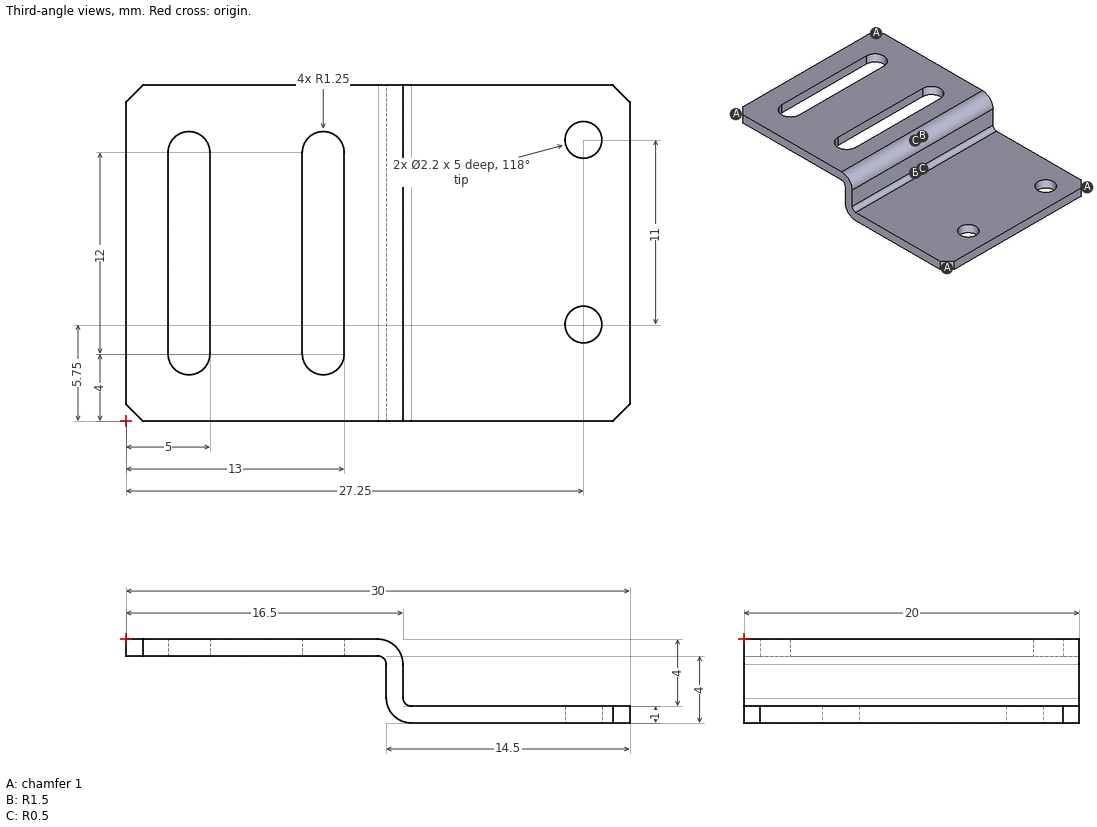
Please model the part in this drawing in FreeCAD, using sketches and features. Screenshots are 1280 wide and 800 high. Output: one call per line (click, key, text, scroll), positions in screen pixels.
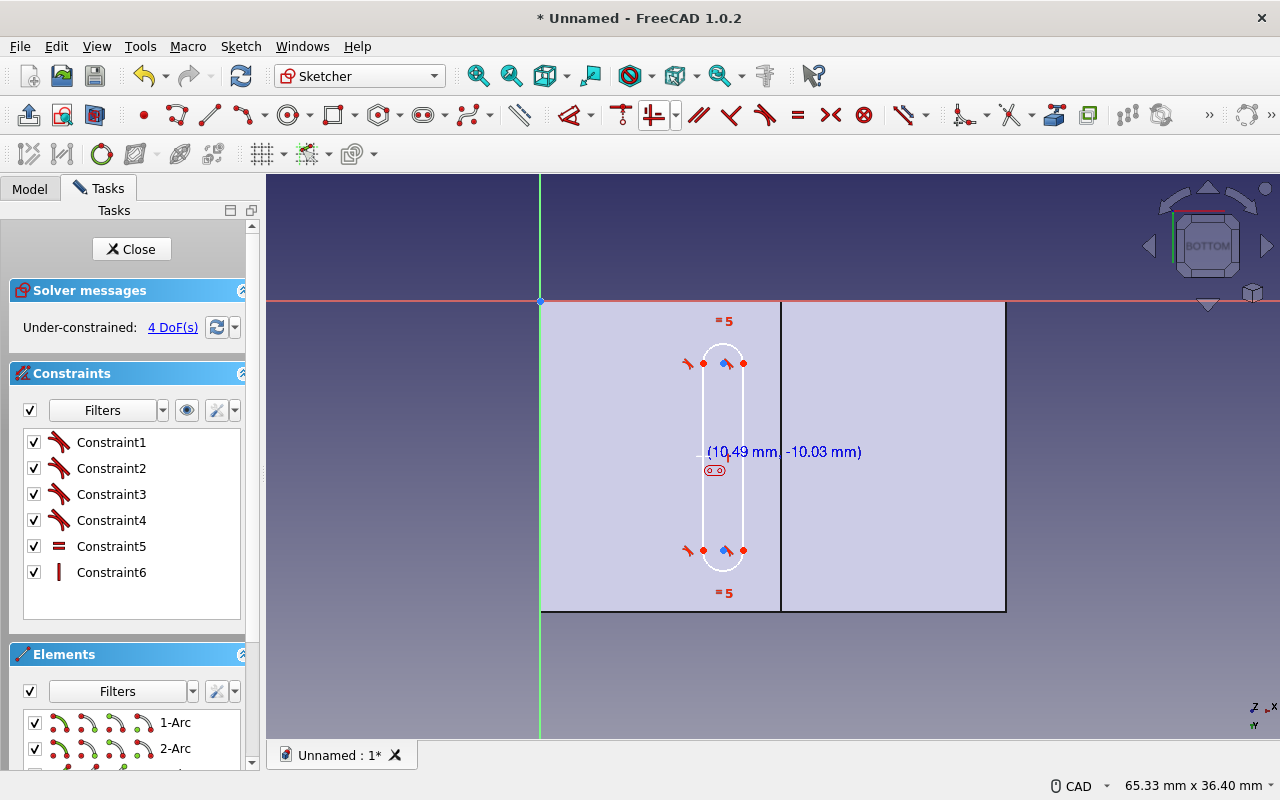
click(598, 550)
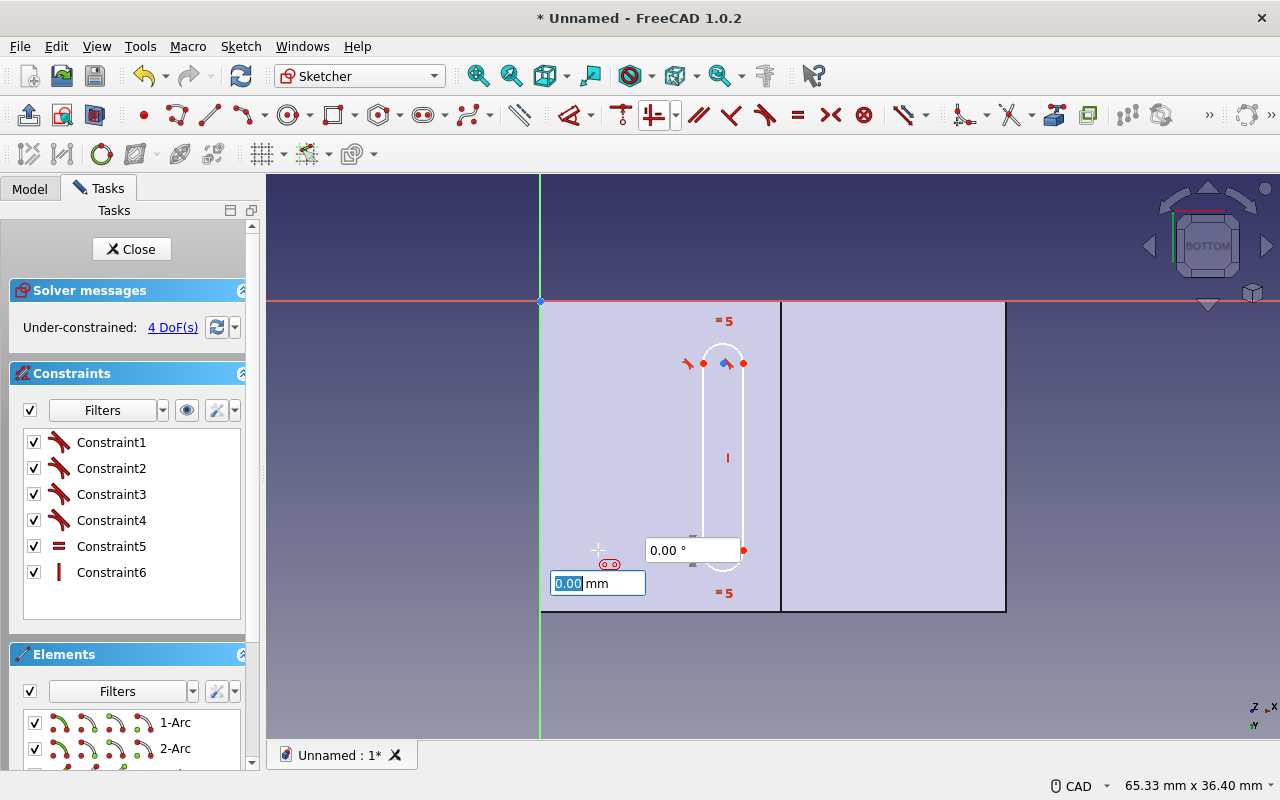
click(598, 363)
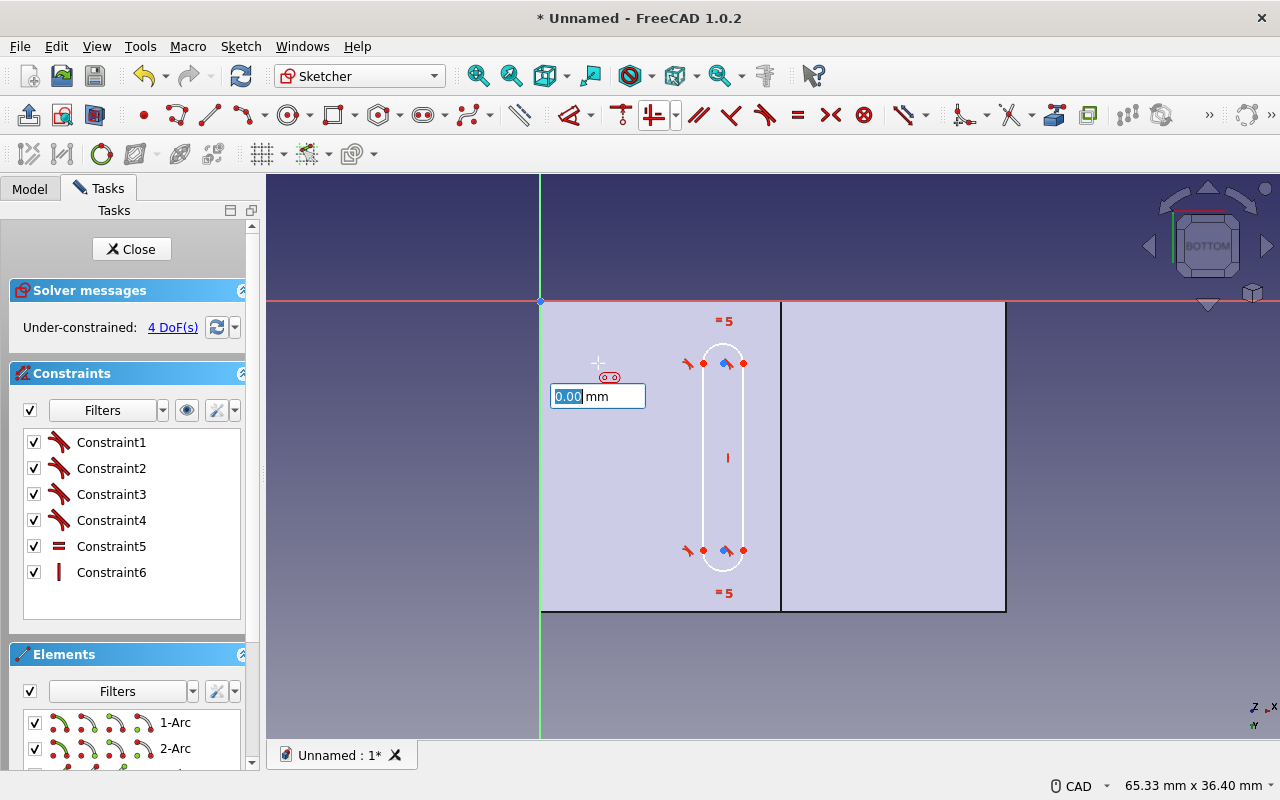
click(618, 456)
key(Escape)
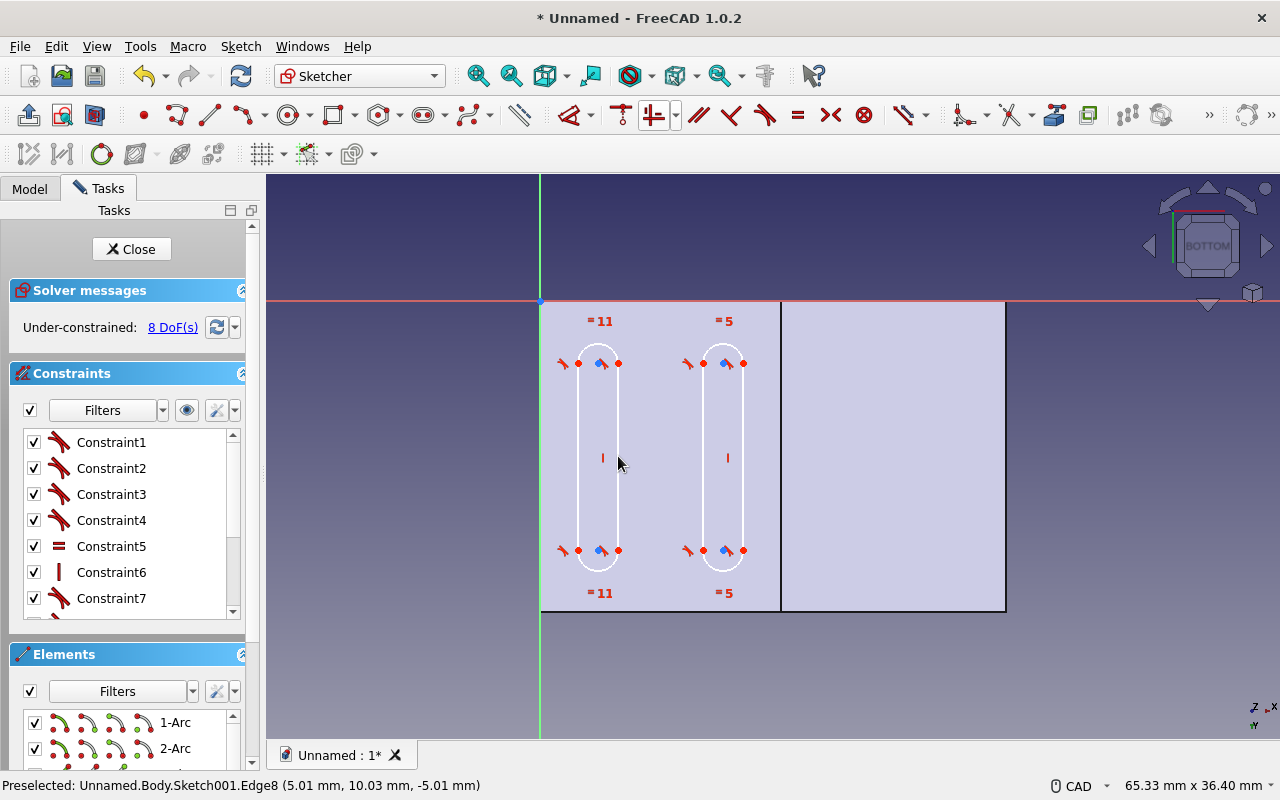
click(711, 567)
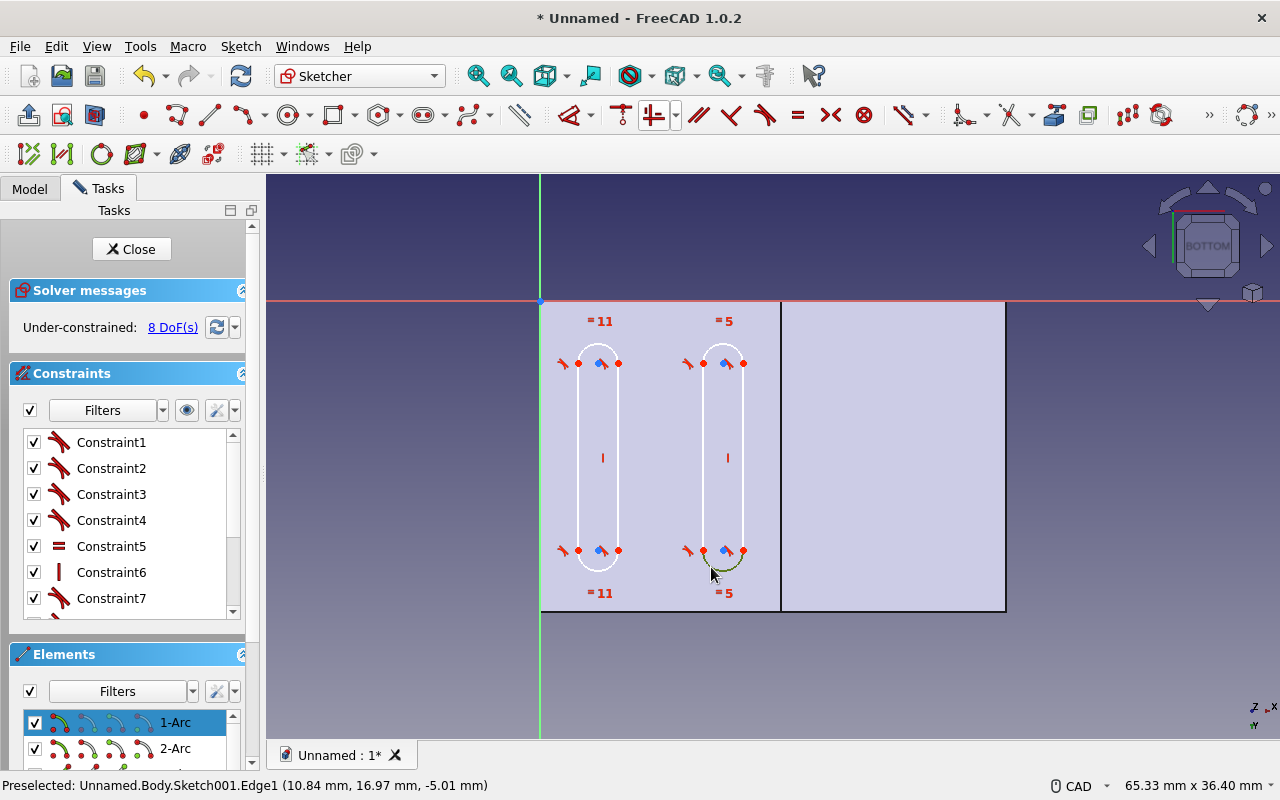
click(586, 567)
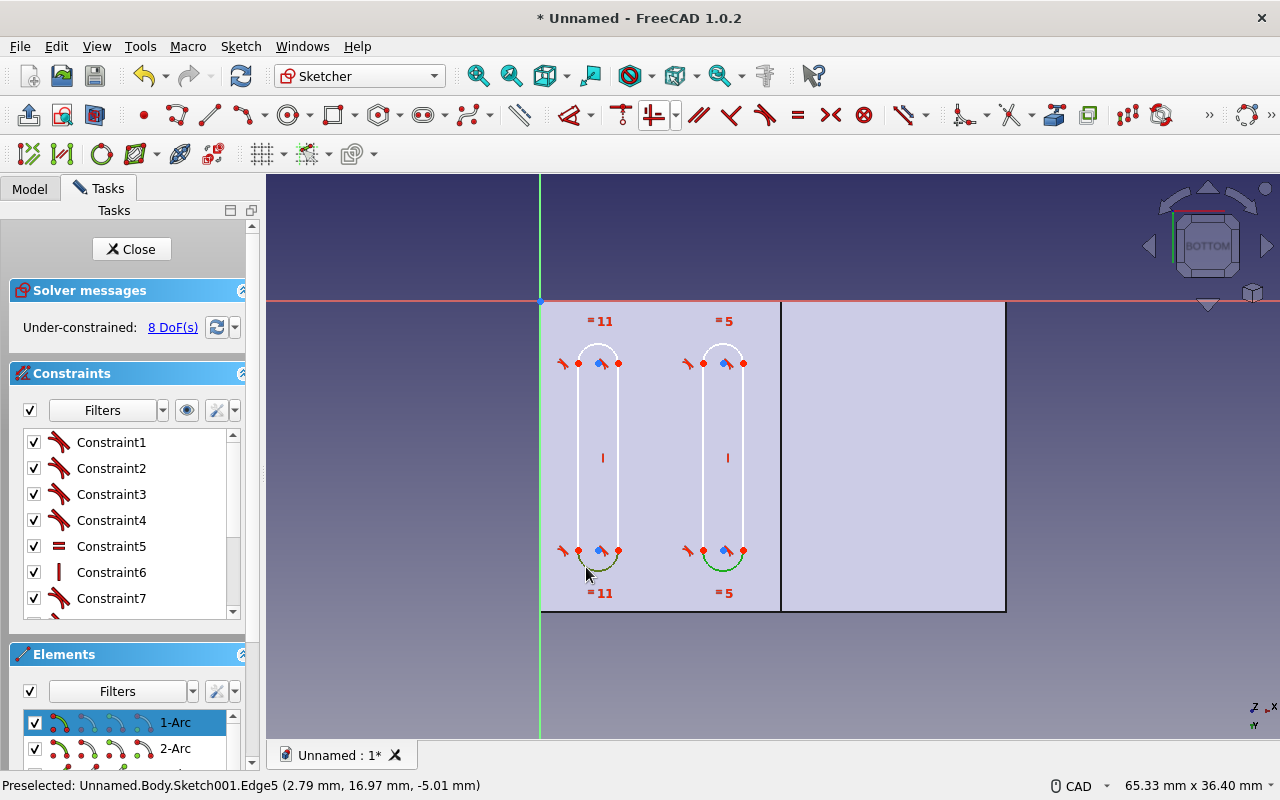
click(798, 116)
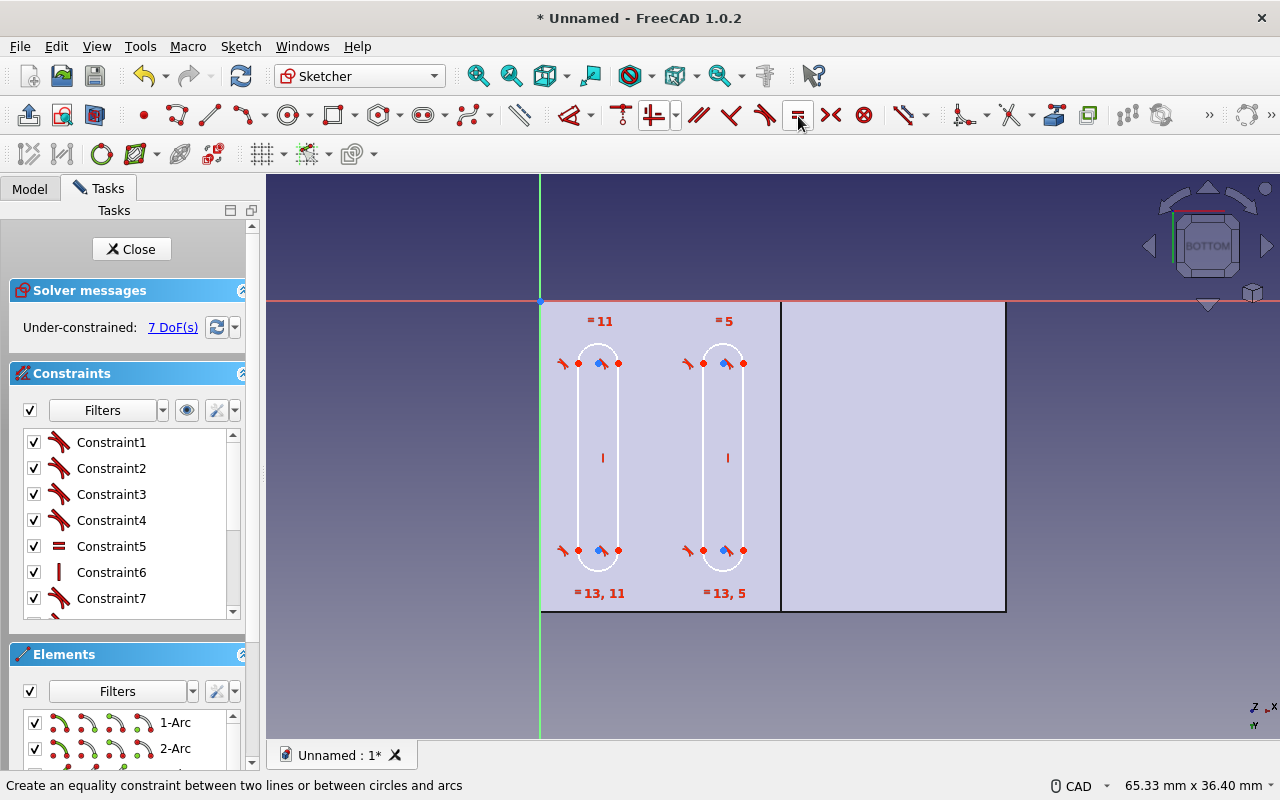
click(568, 116)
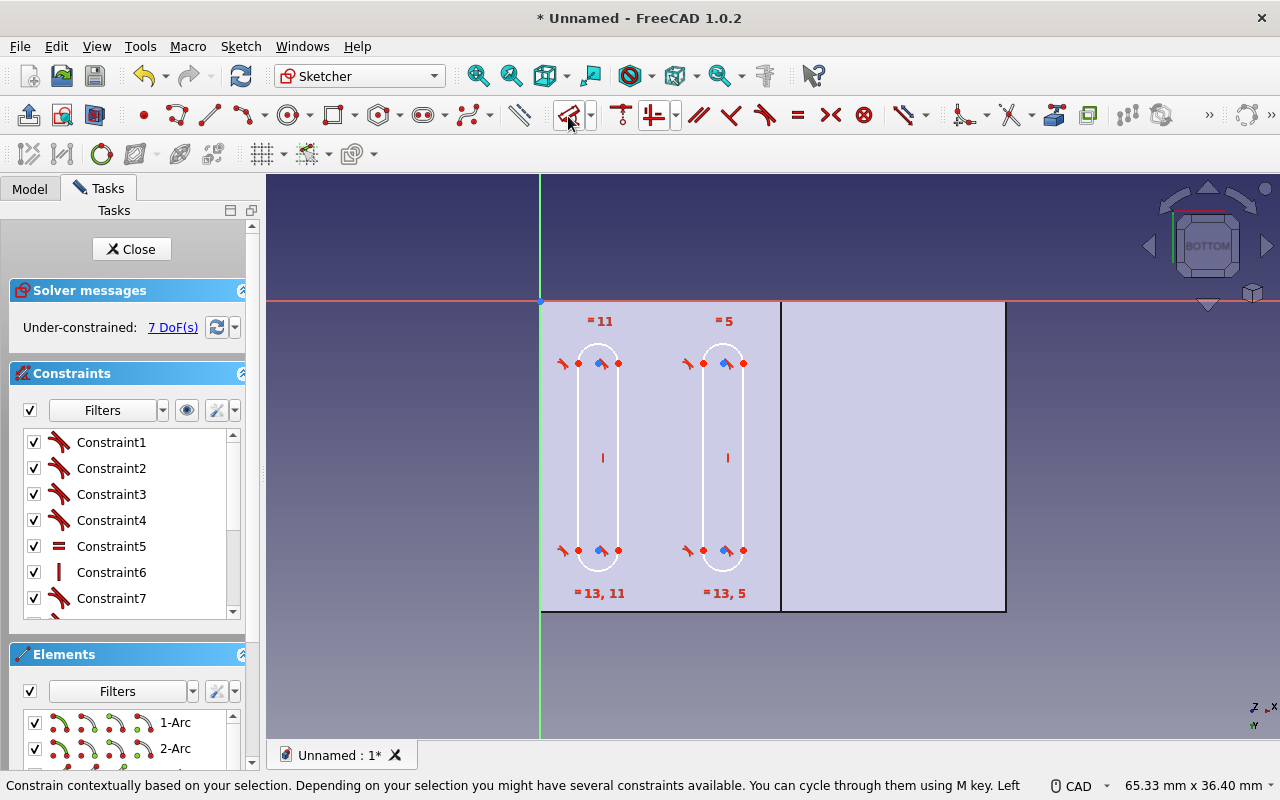
scroll(711, 567, up, 4)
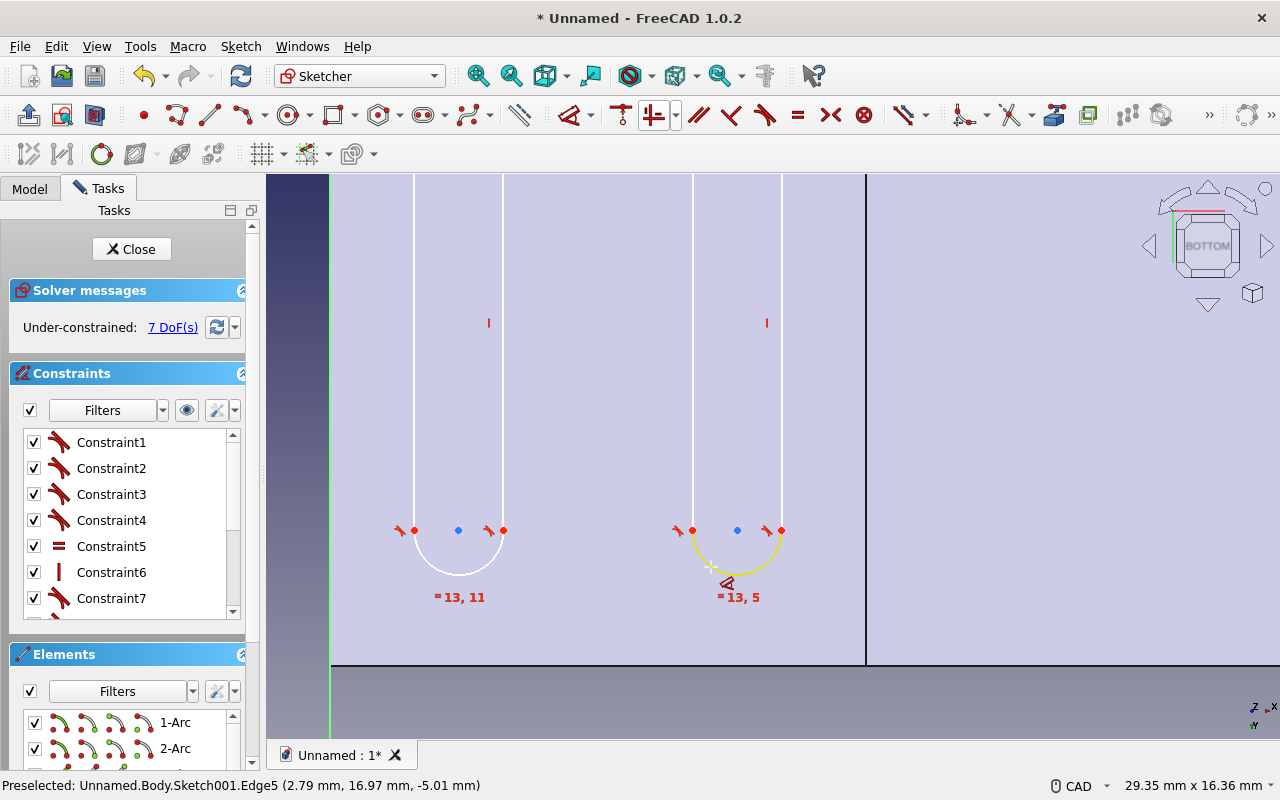
click(711, 567)
click(692, 593)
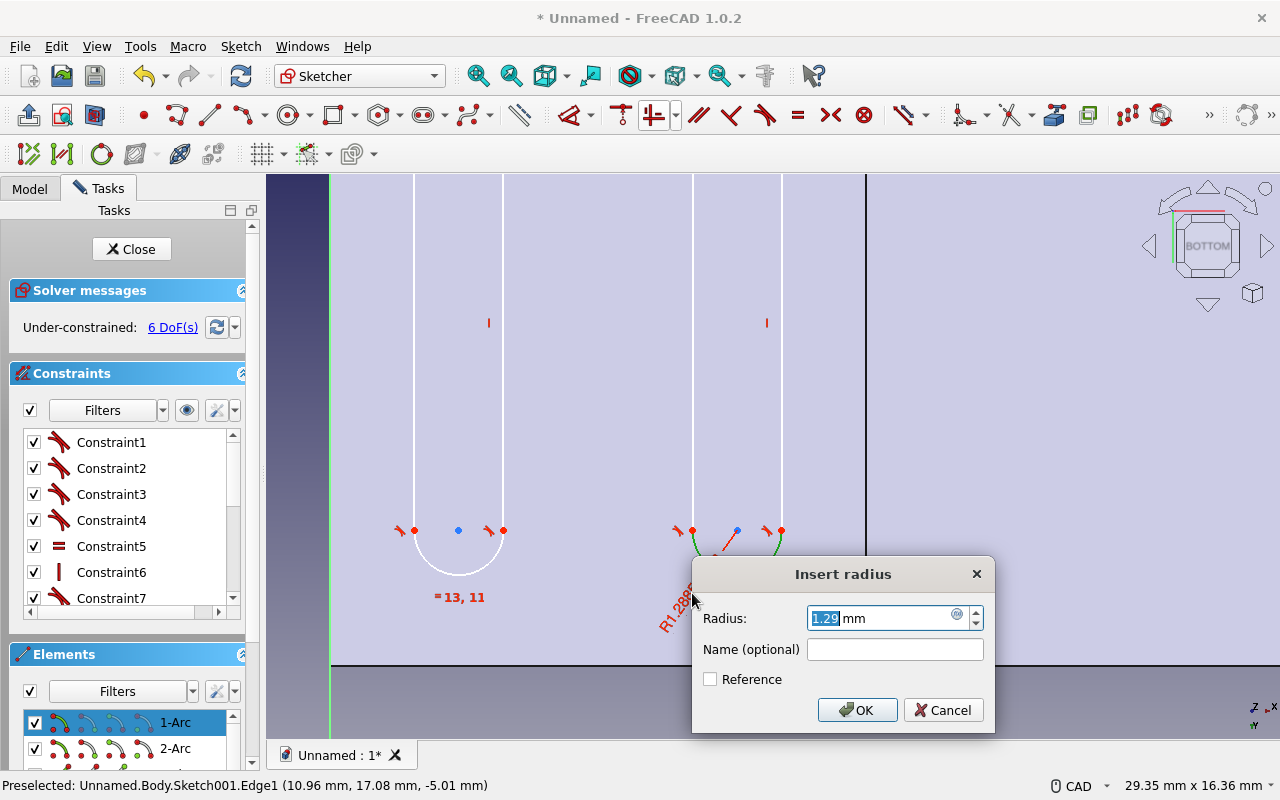
text(1.25)
key(Return)